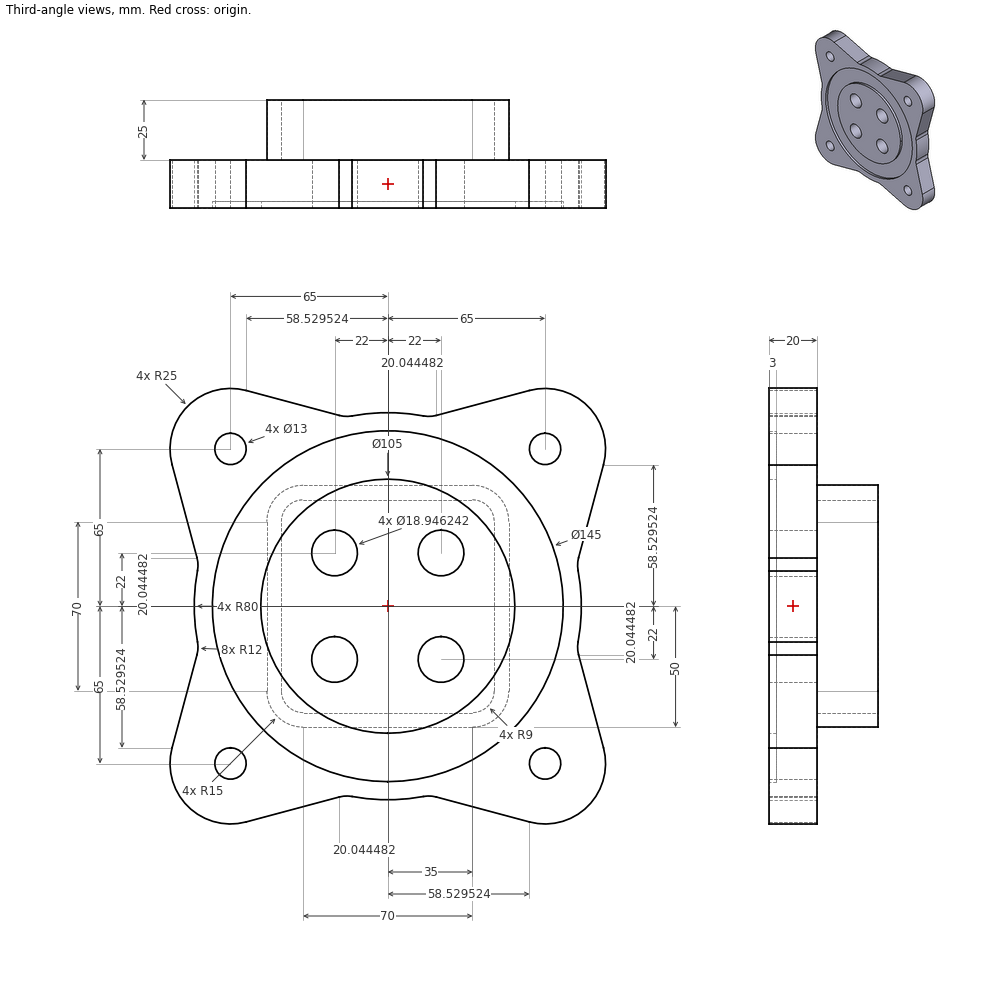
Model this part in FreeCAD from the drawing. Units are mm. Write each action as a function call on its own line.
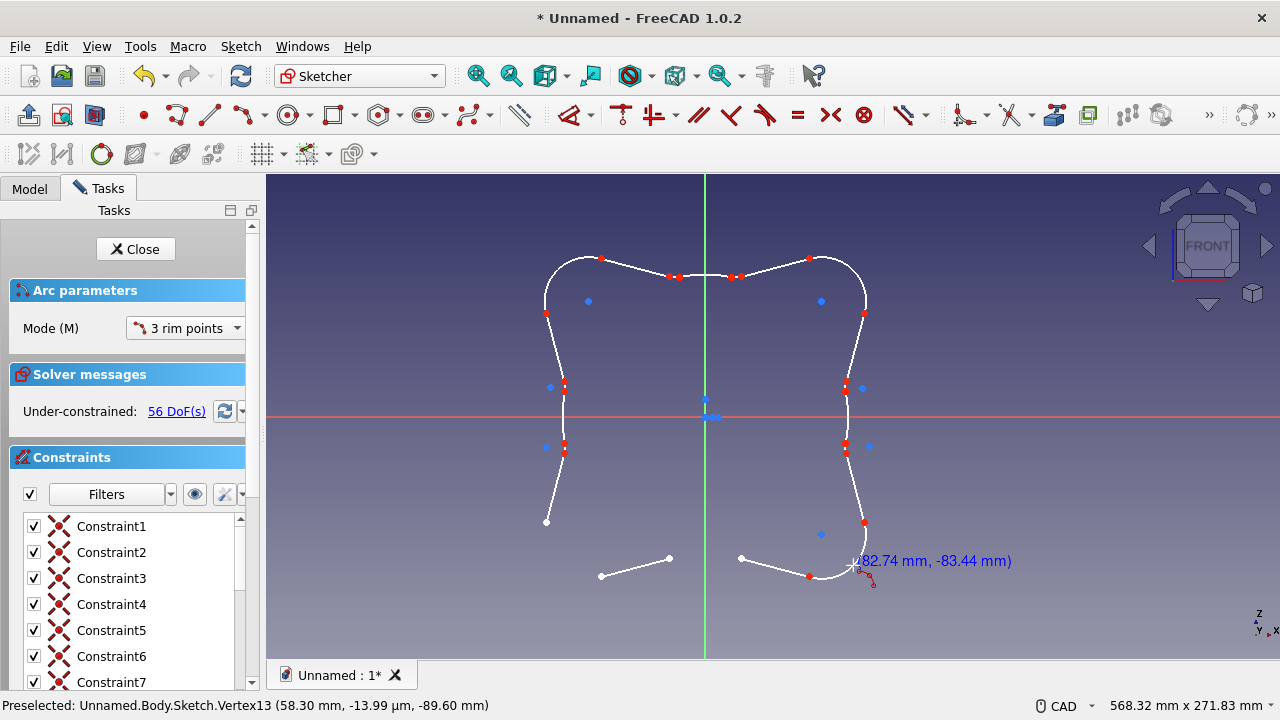
click(741, 559)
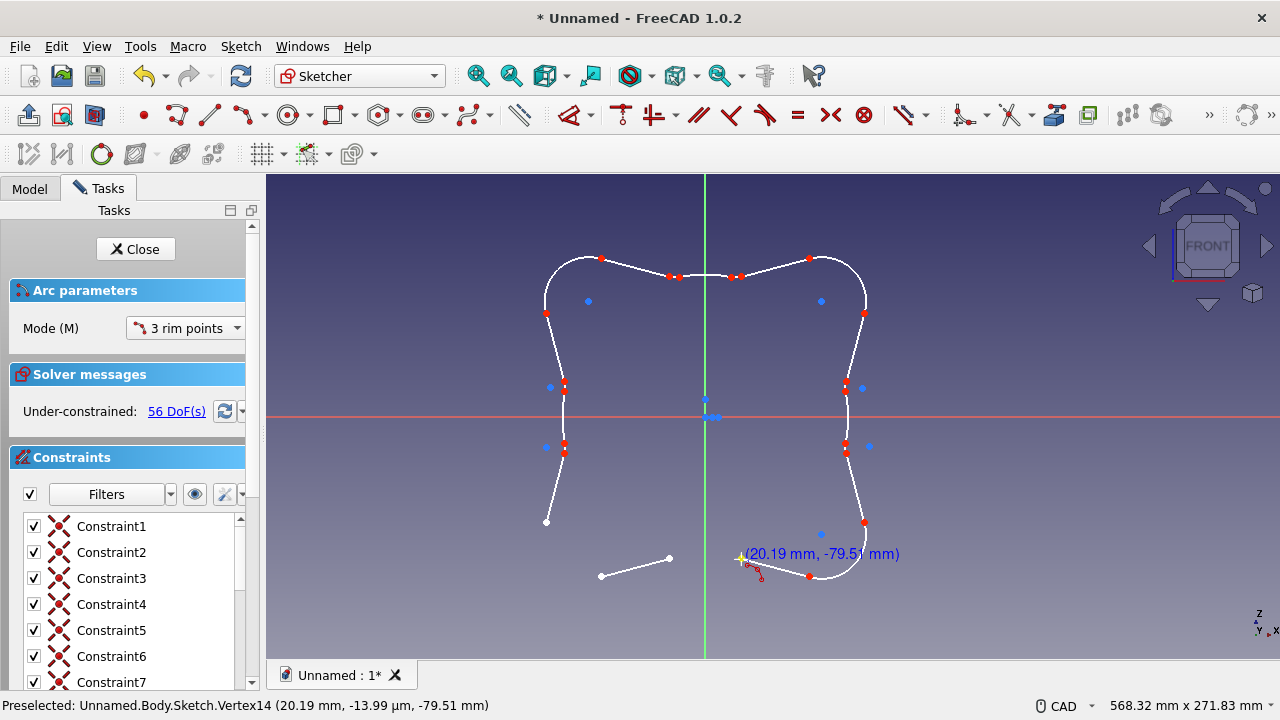
scroll(732, 557, up, 3)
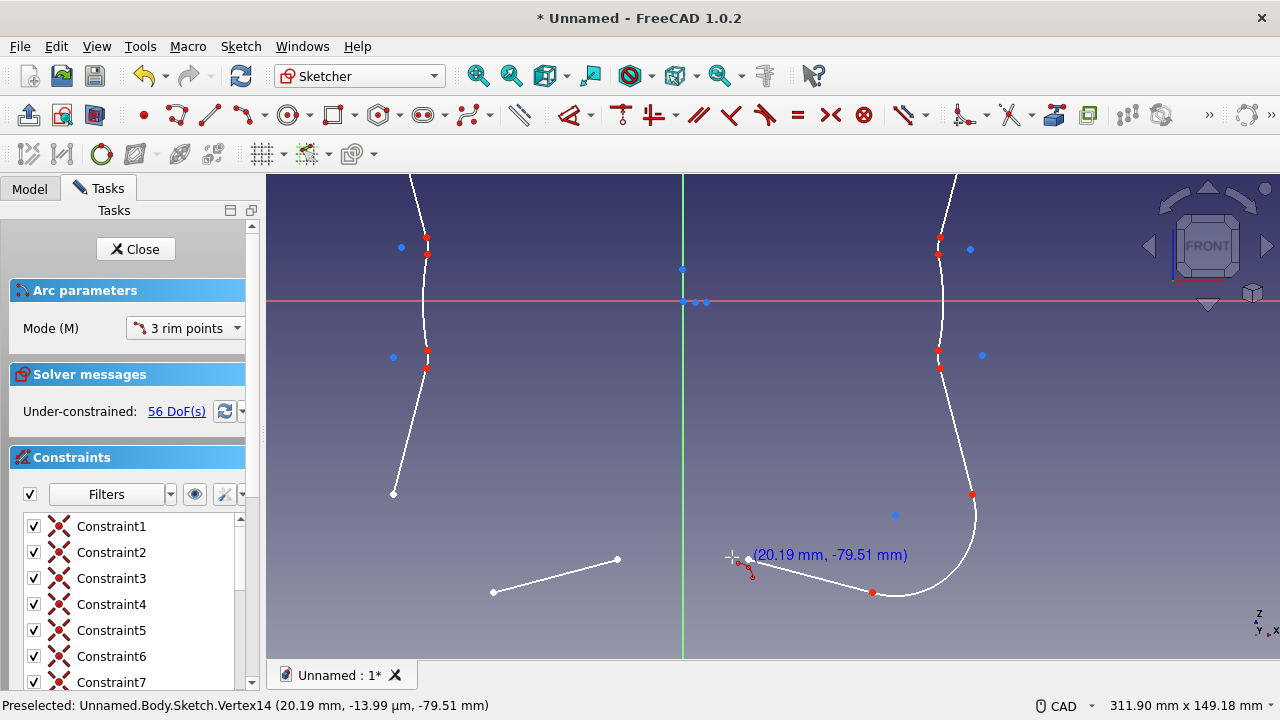
click(731, 557)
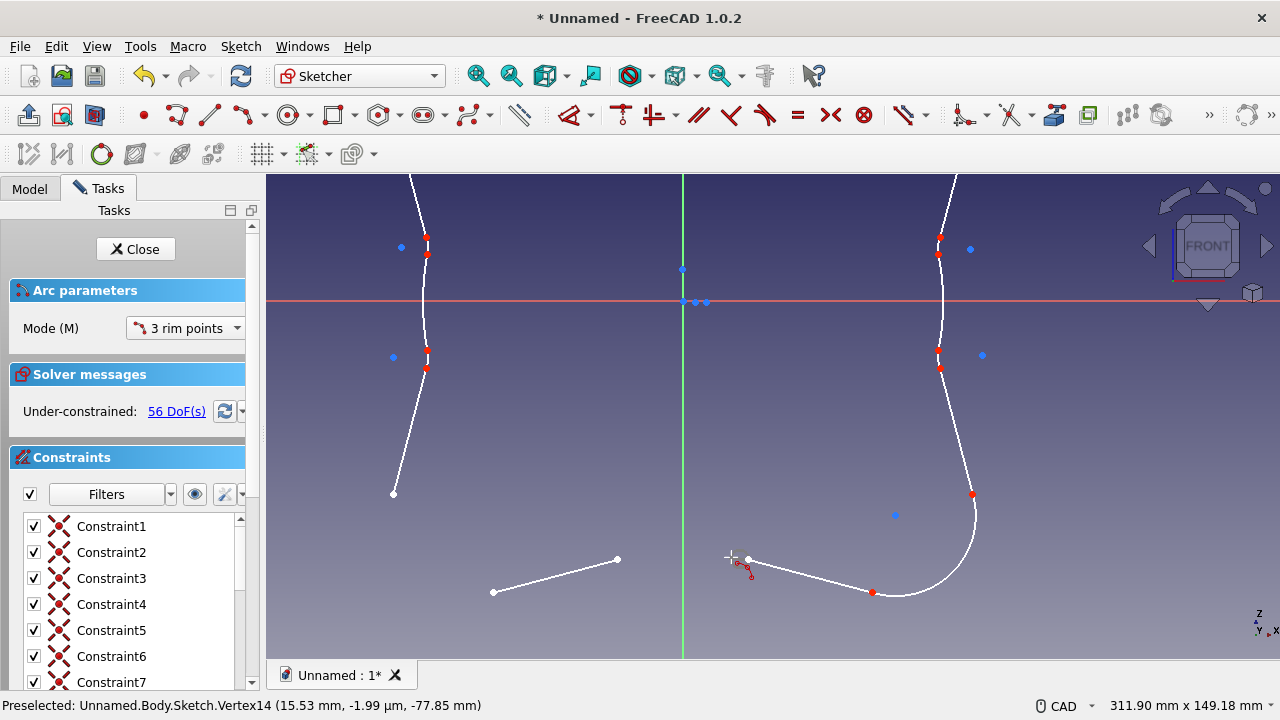
scroll(740, 556, up, 14)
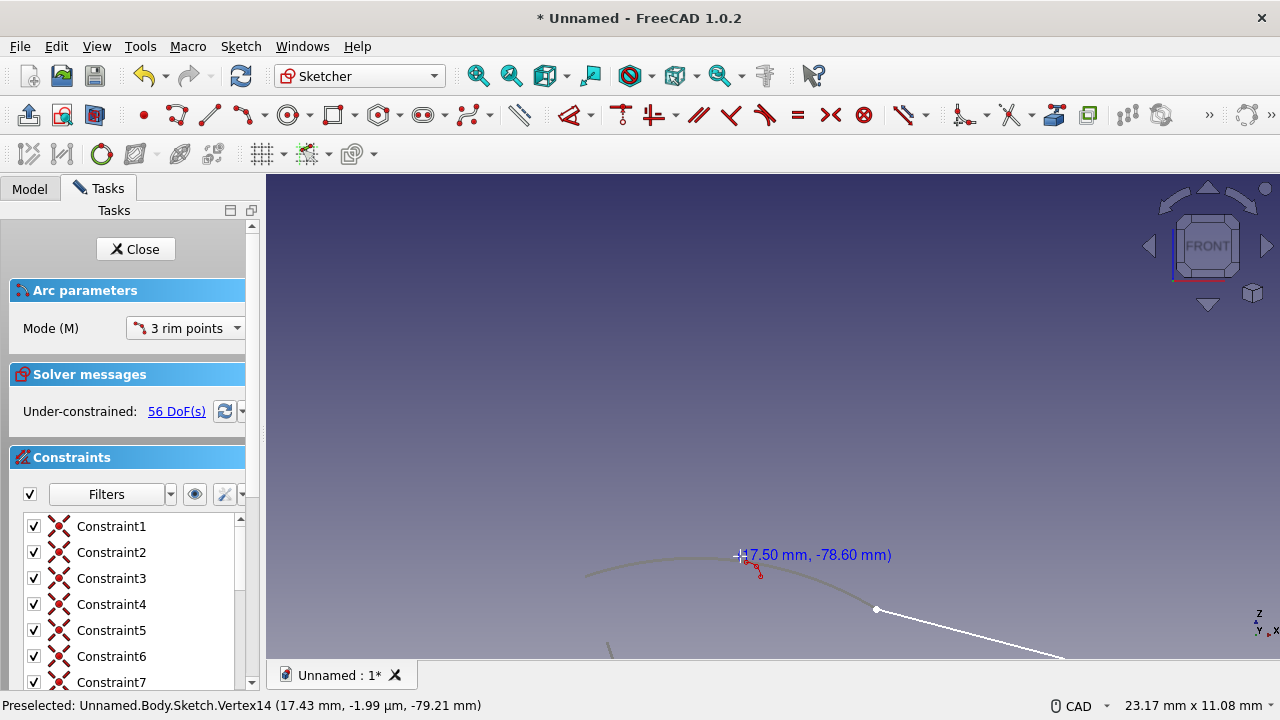
click(727, 552)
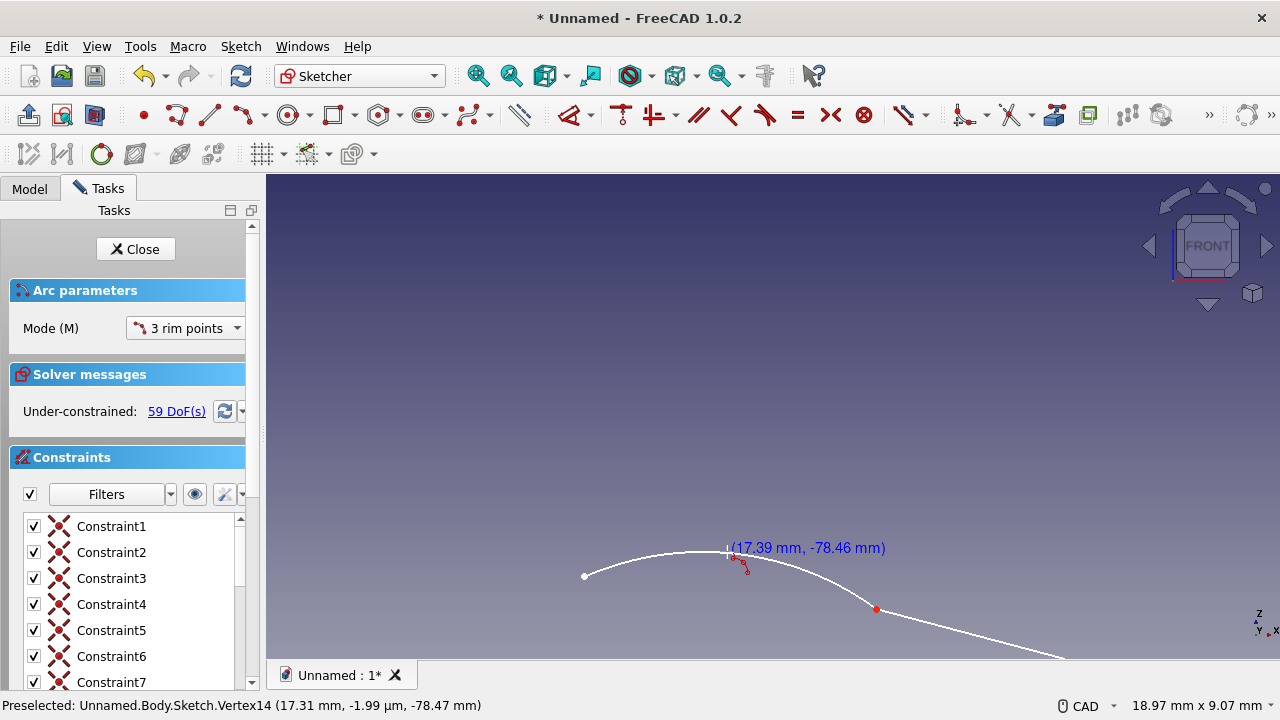
scroll(736, 557, down, 17)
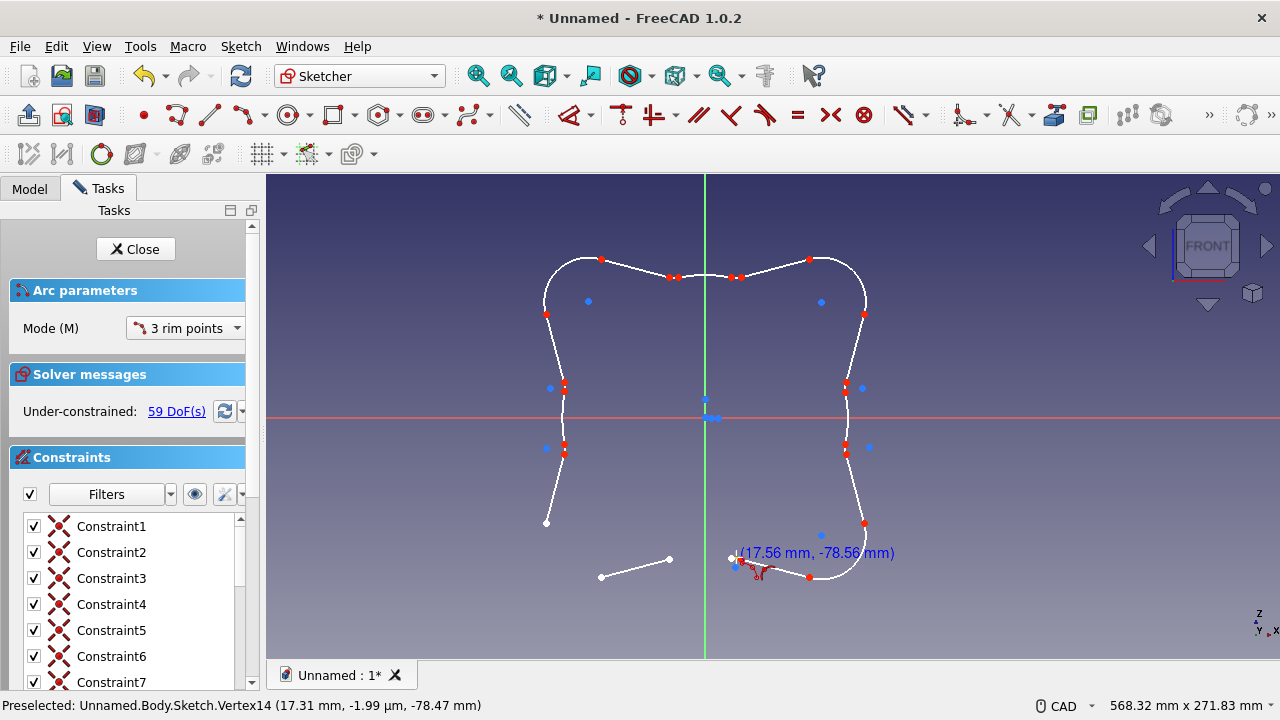
scroll(731, 558, up, 3)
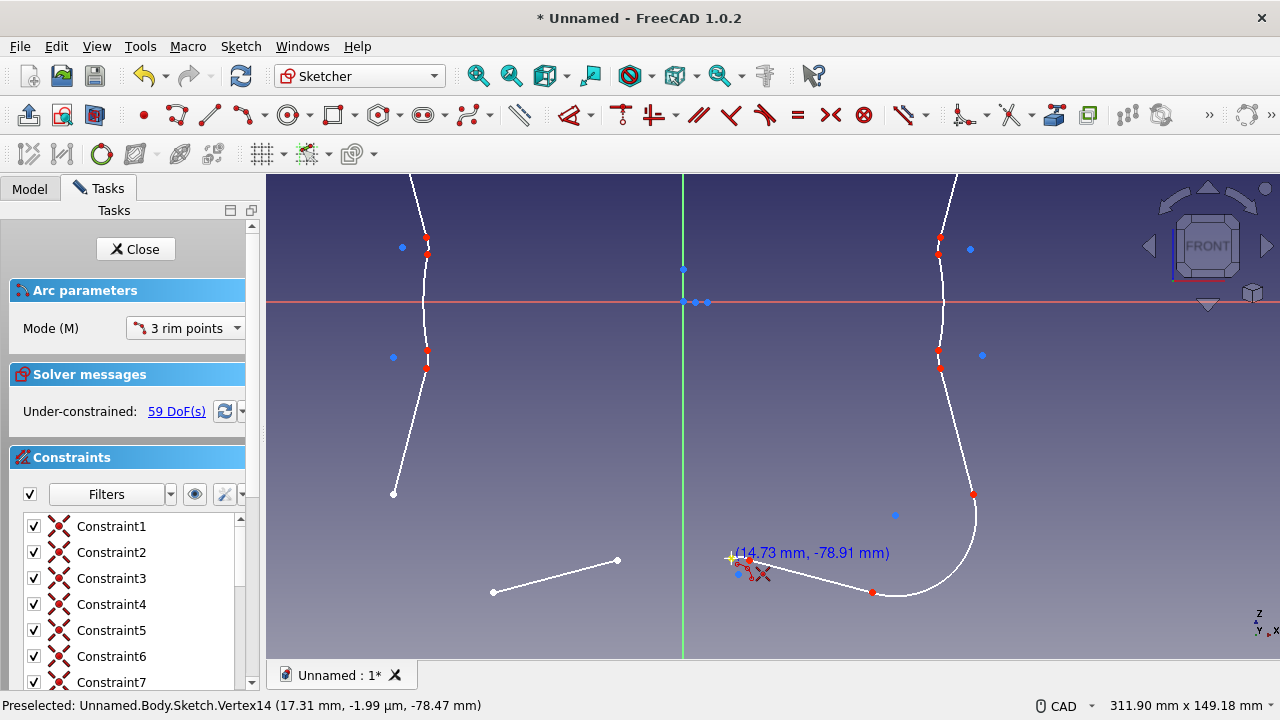
click(731, 558)
click(636, 557)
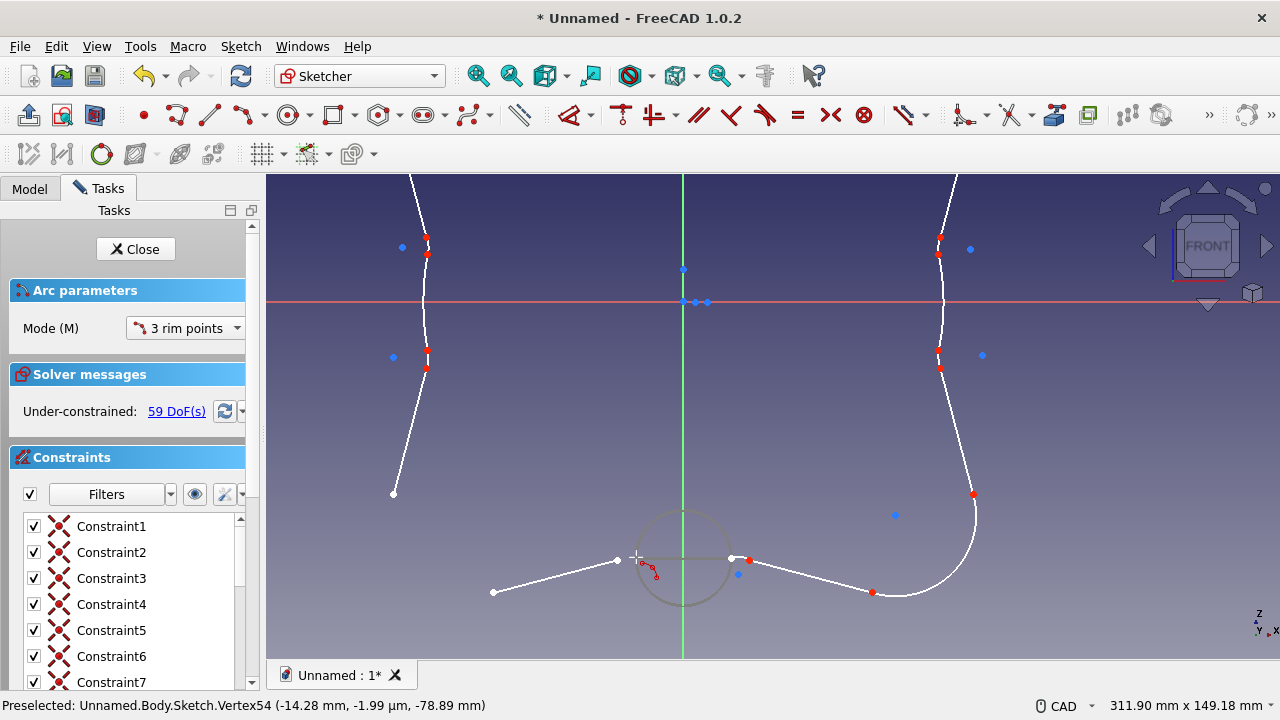
scroll(674, 561, up, 7)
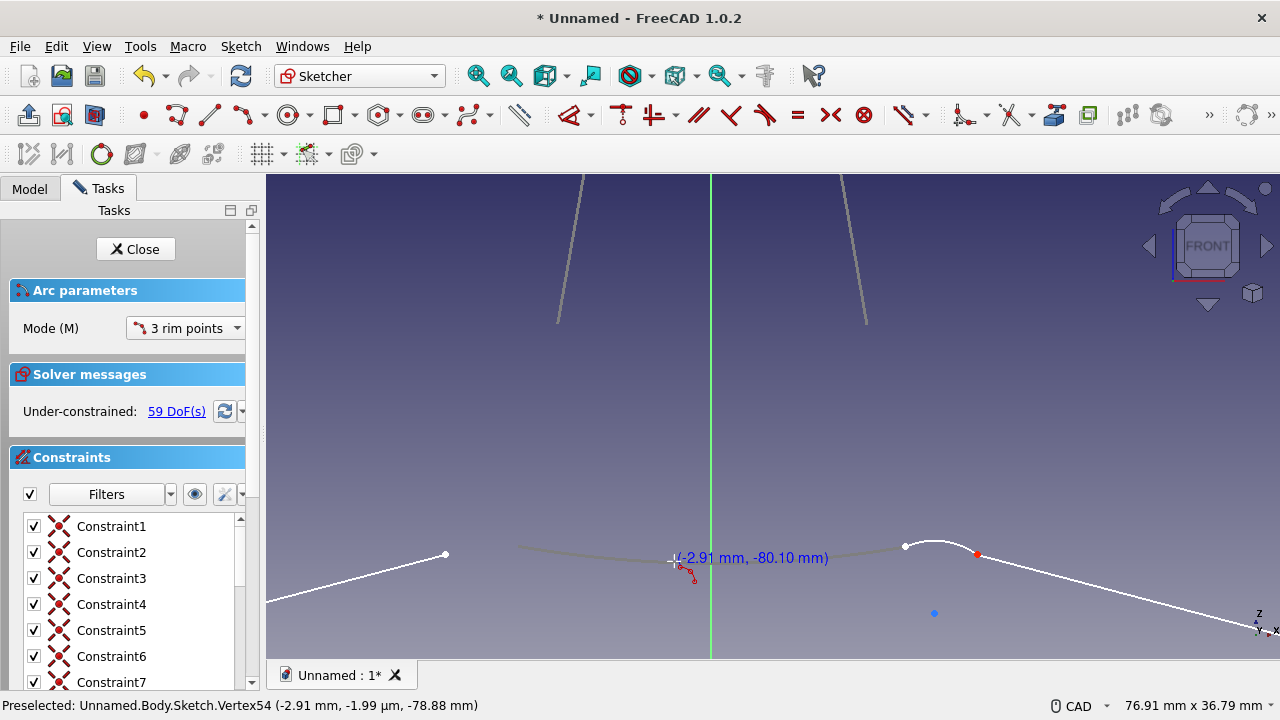
click(672, 561)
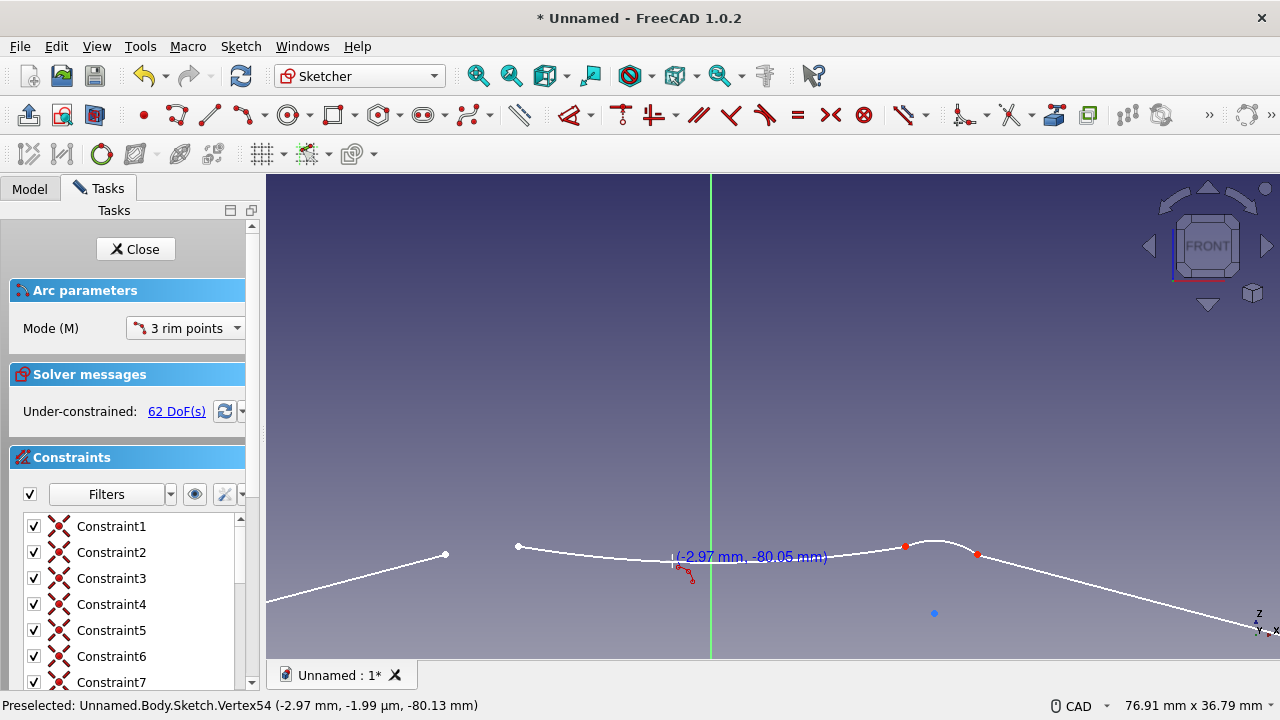
scroll(703, 559, down, 10)